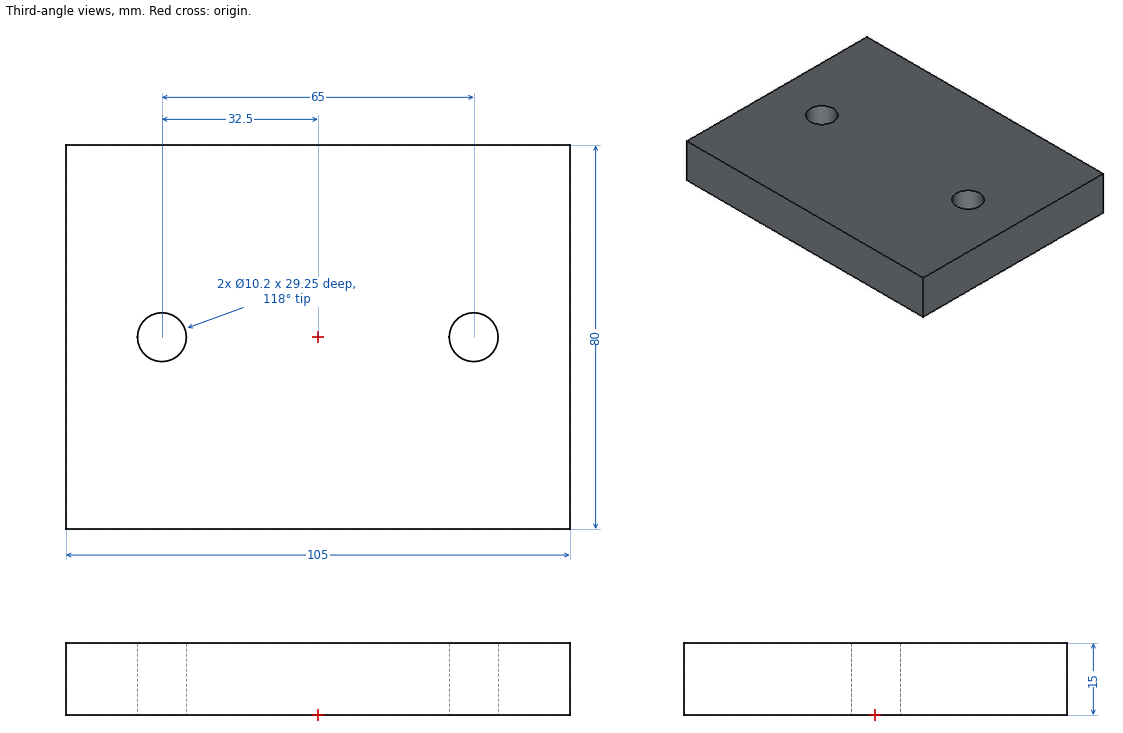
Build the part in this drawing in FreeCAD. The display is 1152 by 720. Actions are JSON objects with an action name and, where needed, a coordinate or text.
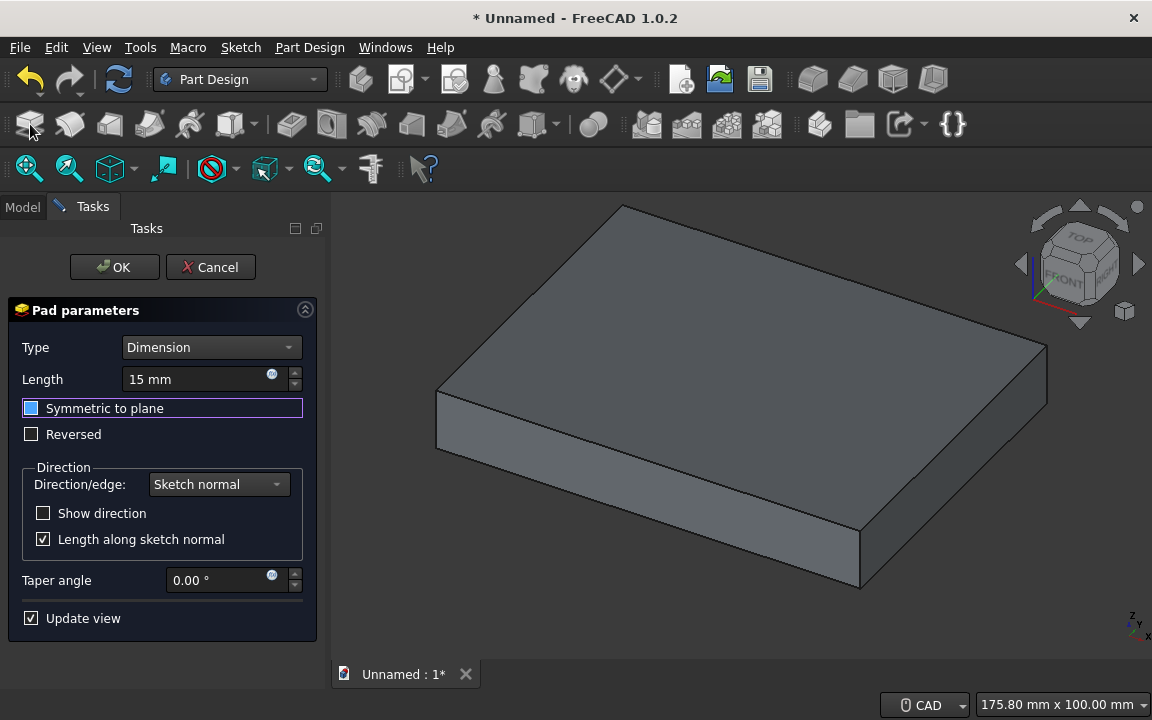
{"action": "left_click", "coordinate": [115, 267]}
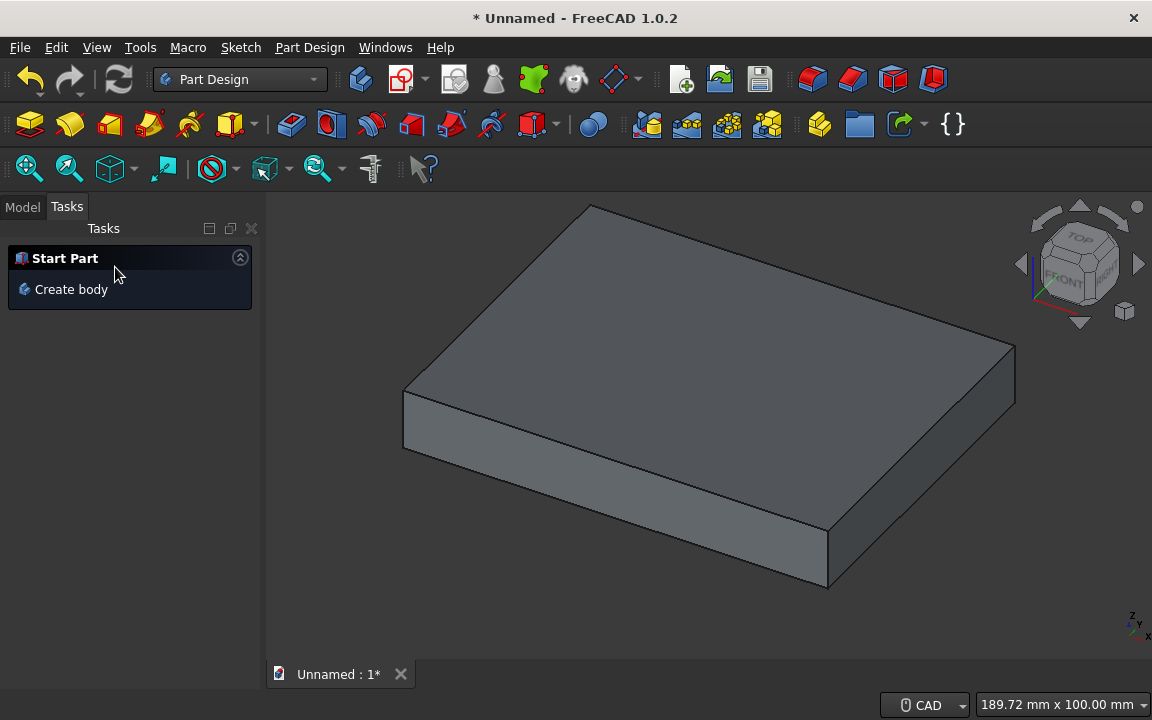
{"action": "left_click", "coordinate": [709, 367]}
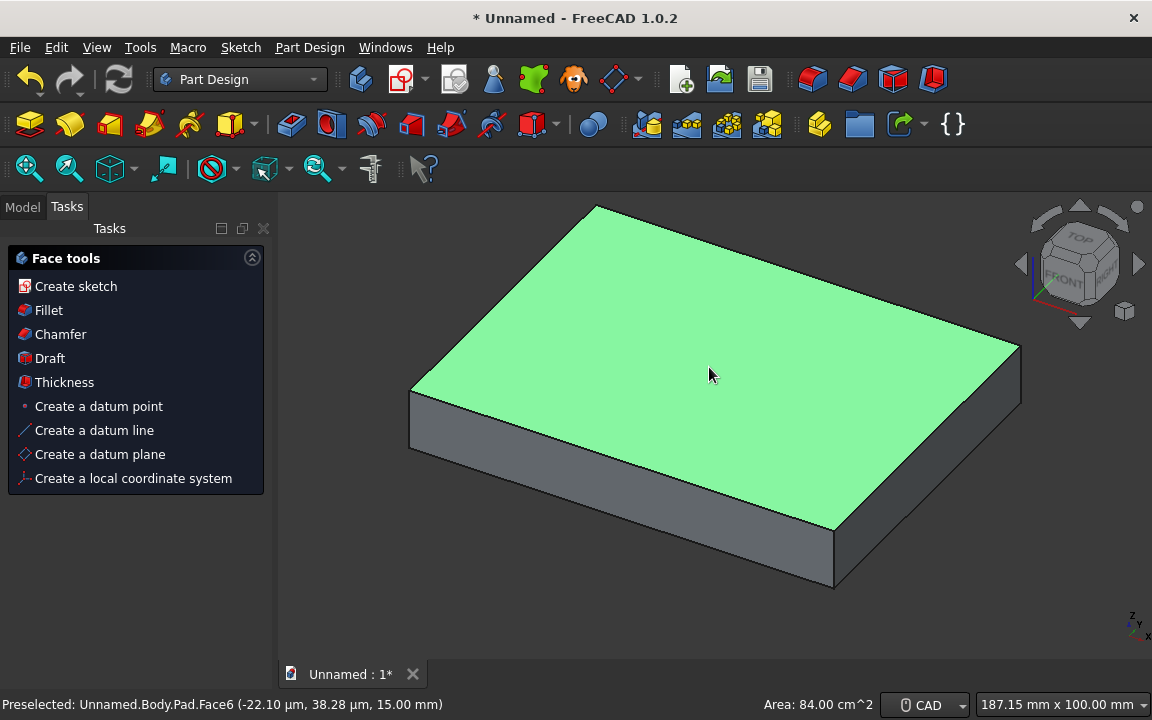
{"action": "left_click", "coordinate": [402, 80]}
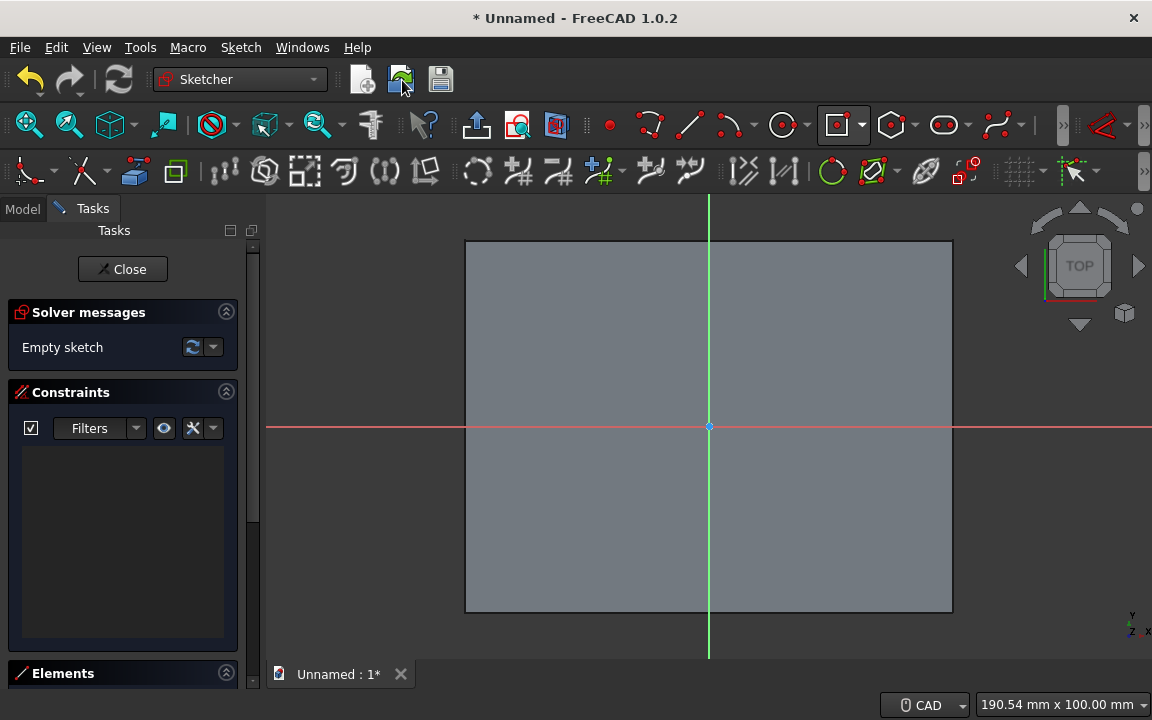
{"action": "scroll", "coordinate": [848, 426], "scroll_direction": "up", "scroll_amount": 2}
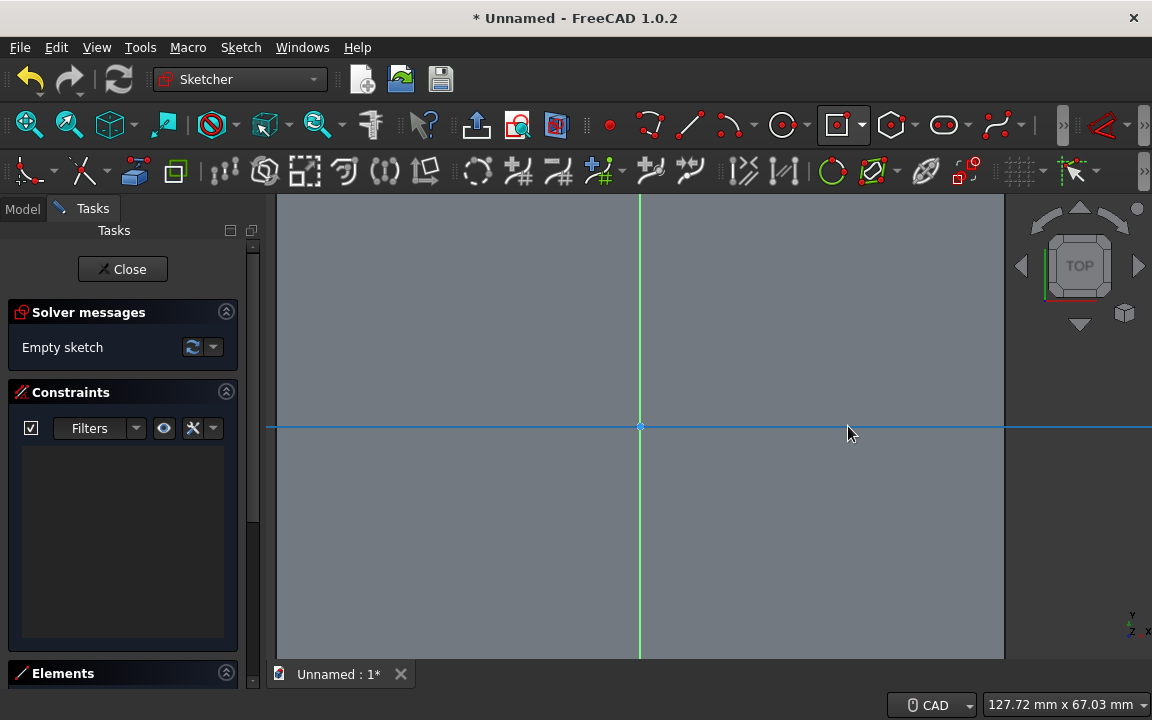
{"action": "left_click", "coordinate": [784, 126]}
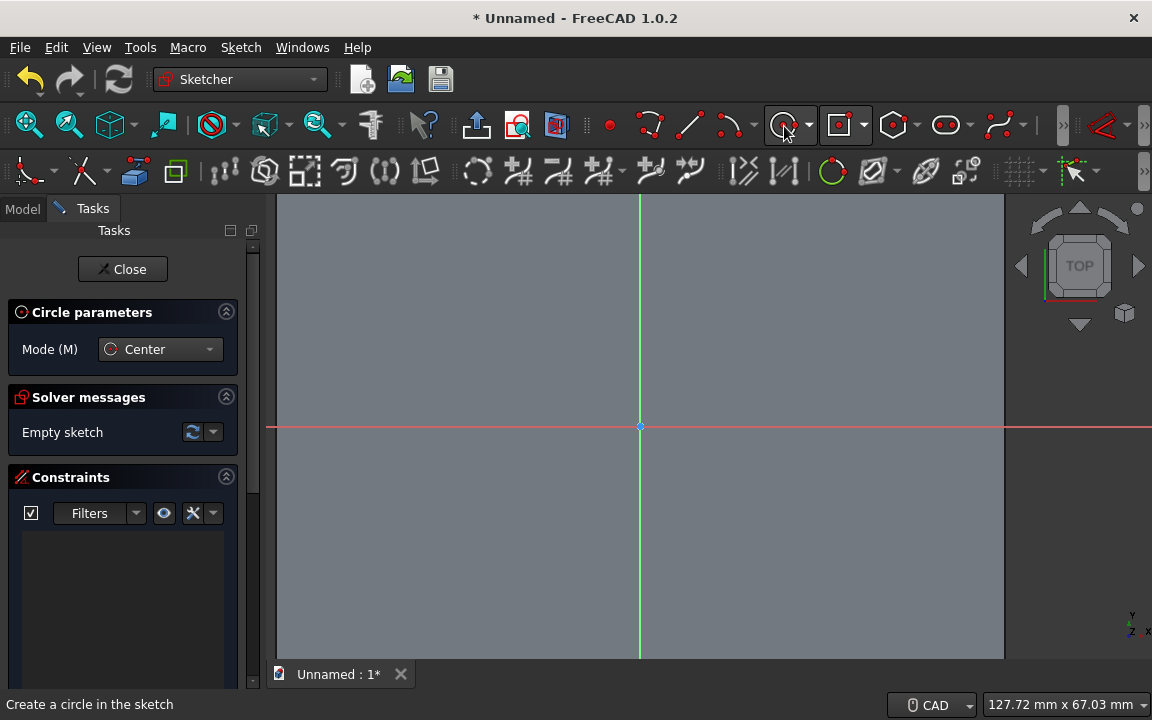
{"action": "left_click", "coordinate": [415, 426]}
{"action": "mouse_move", "coordinate": [440, 401]}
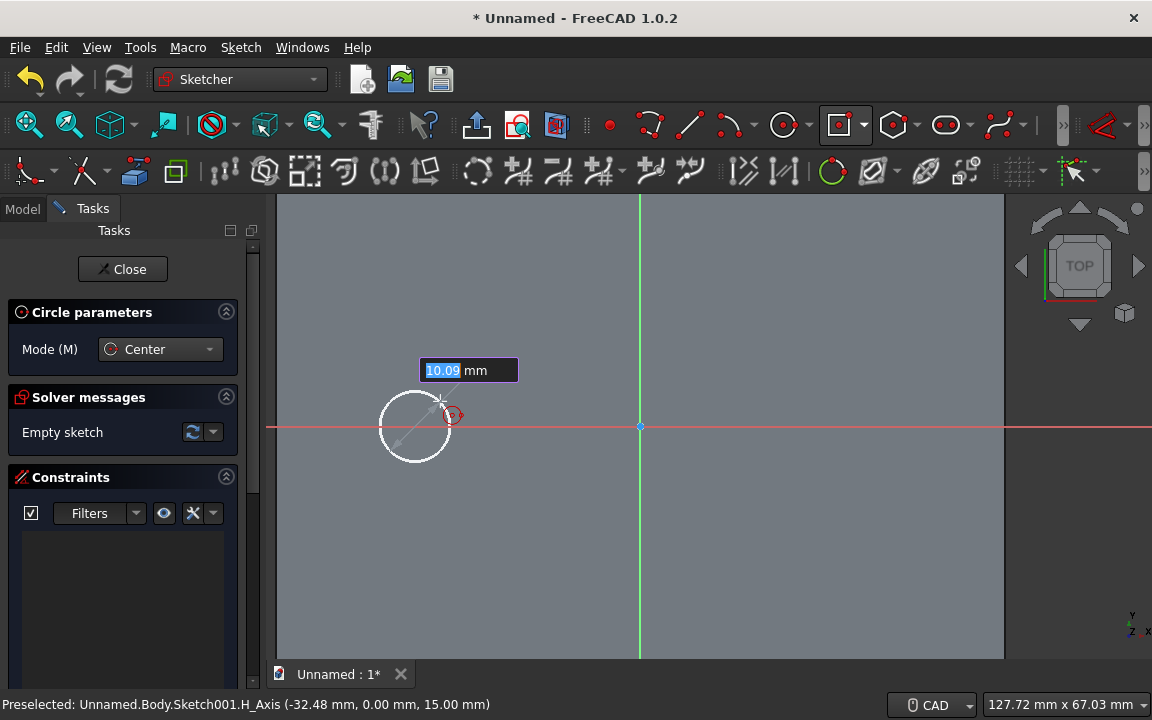
{"action": "type", "text": "10.2"}
{"action": "key", "text": "Return"}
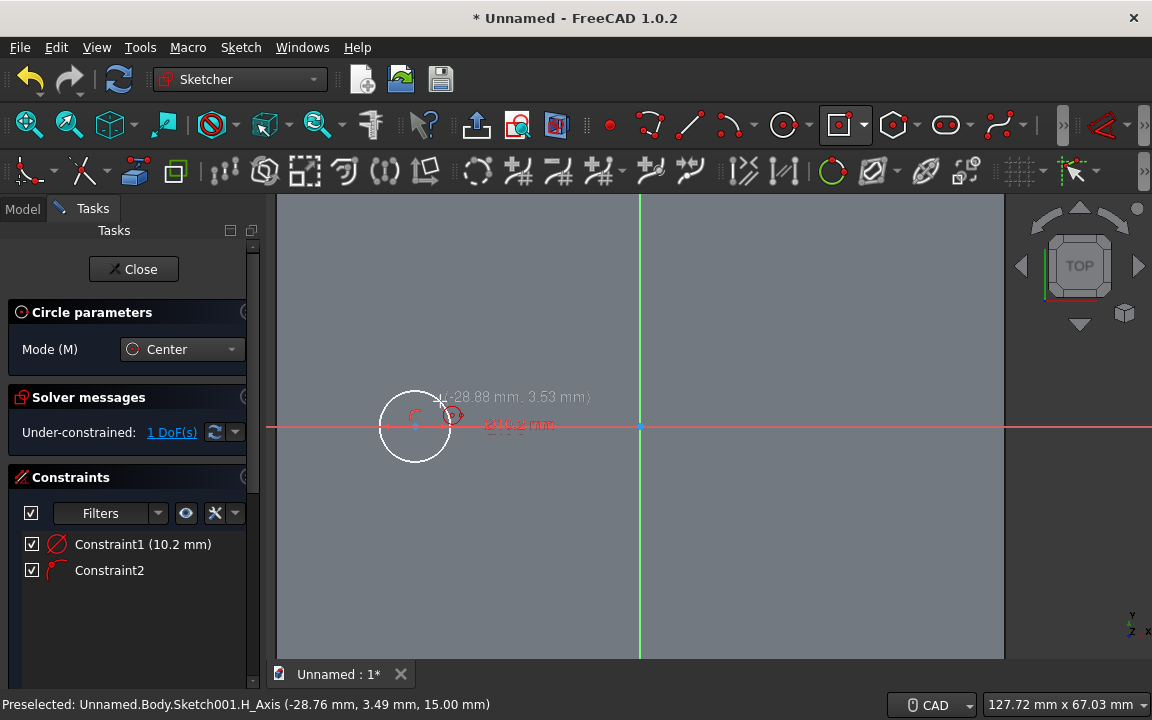
{"action": "left_click", "coordinate": [866, 426]}
{"action": "mouse_move", "coordinate": [891, 401]}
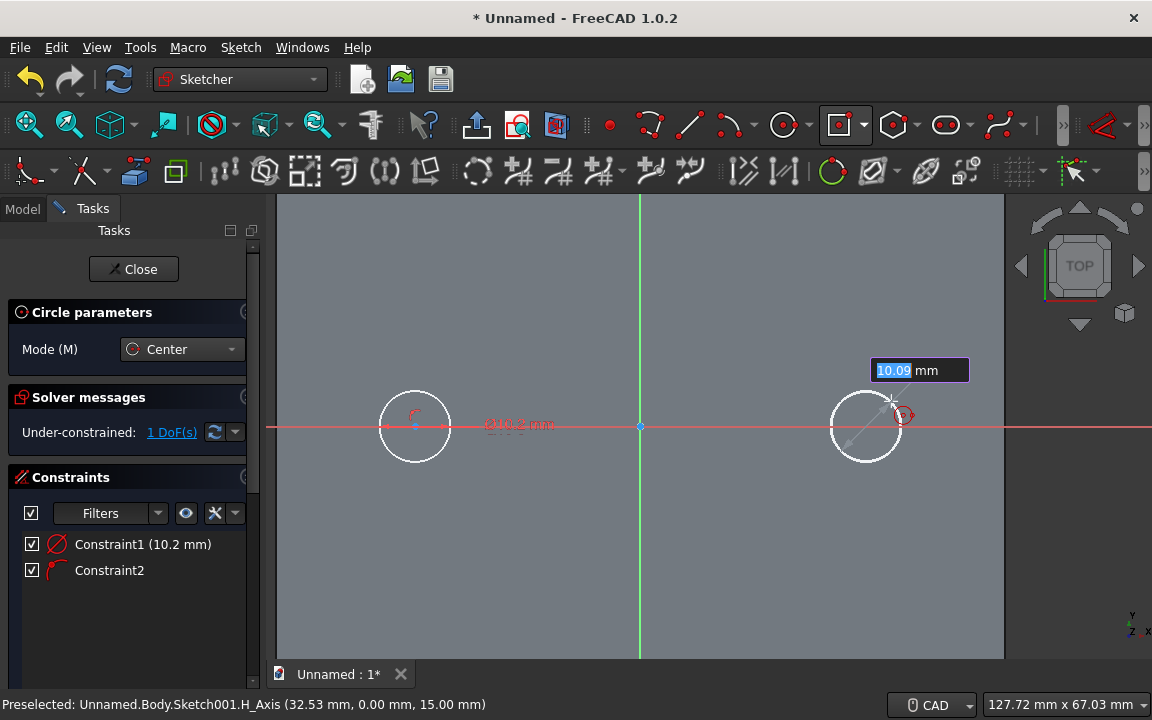
{"action": "type", "text": "10.2"}
{"action": "key", "text": "Return"}
{"action": "key", "text": "Escape"}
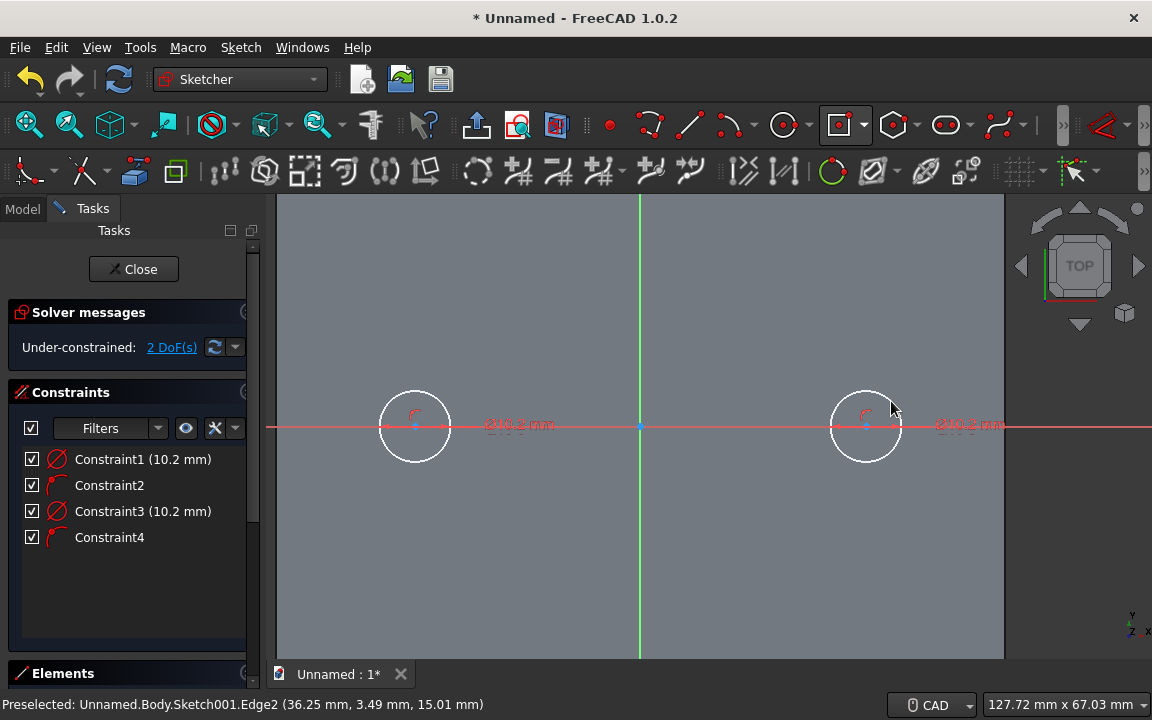
{"action": "left_click", "coordinate": [415, 426]}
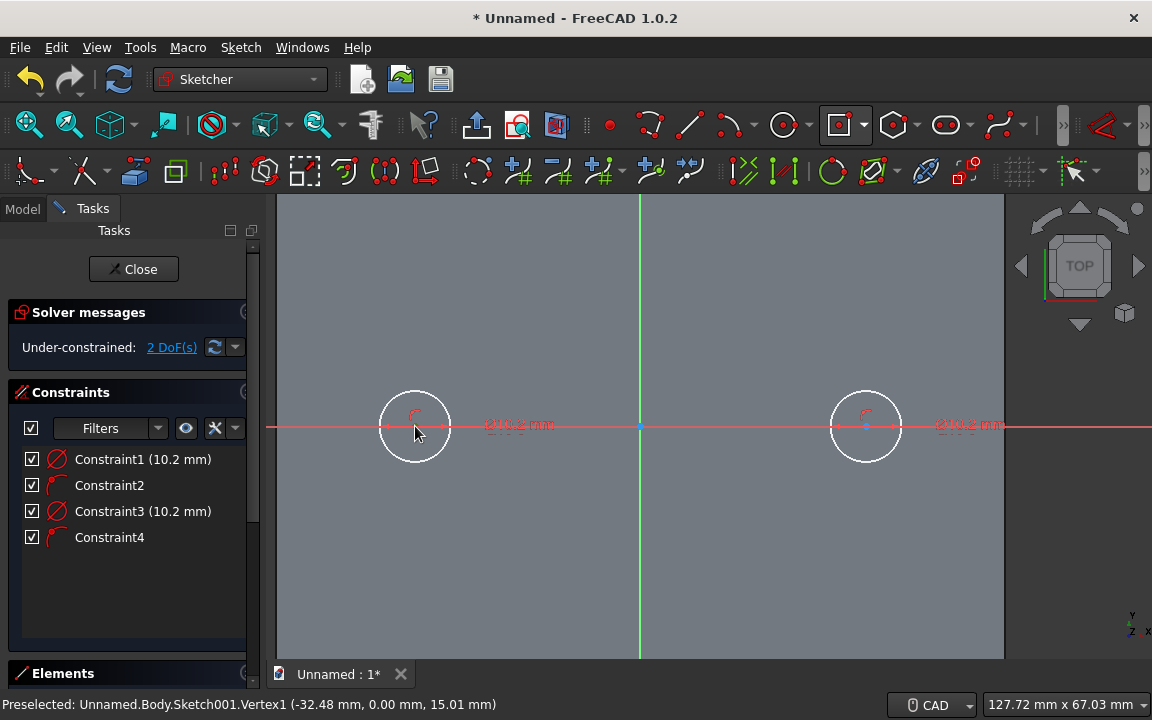
{"action": "left_click", "coordinate": [866, 426]}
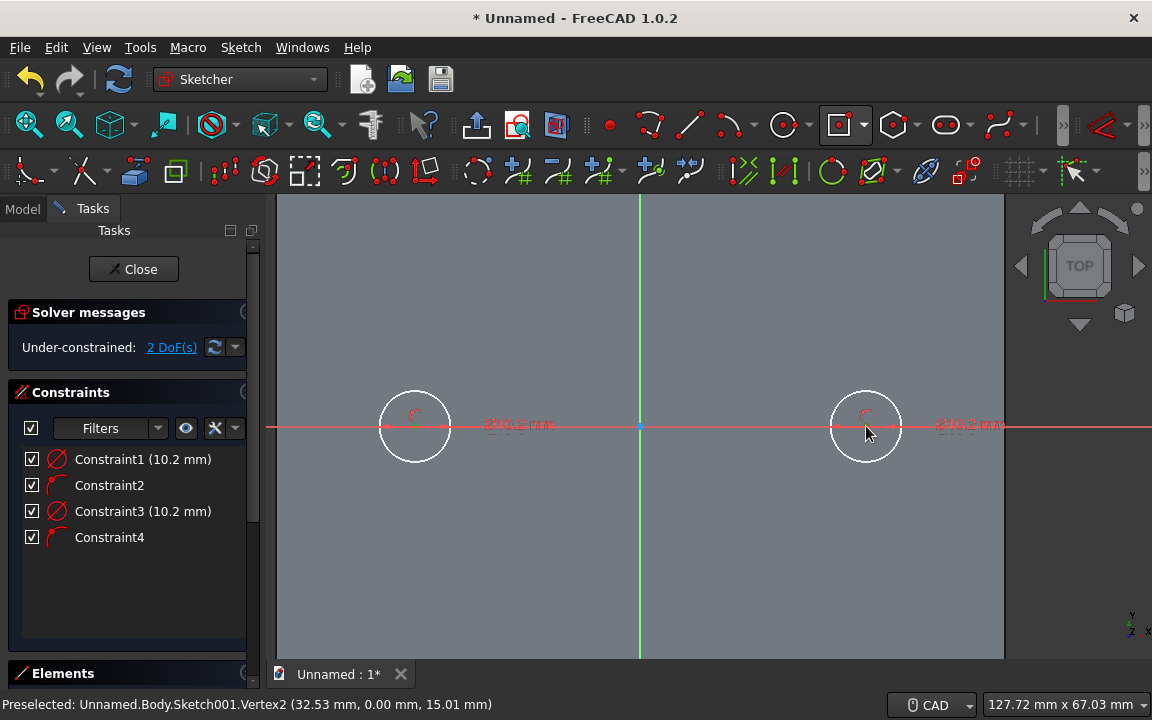
{"action": "key", "text": "l"}